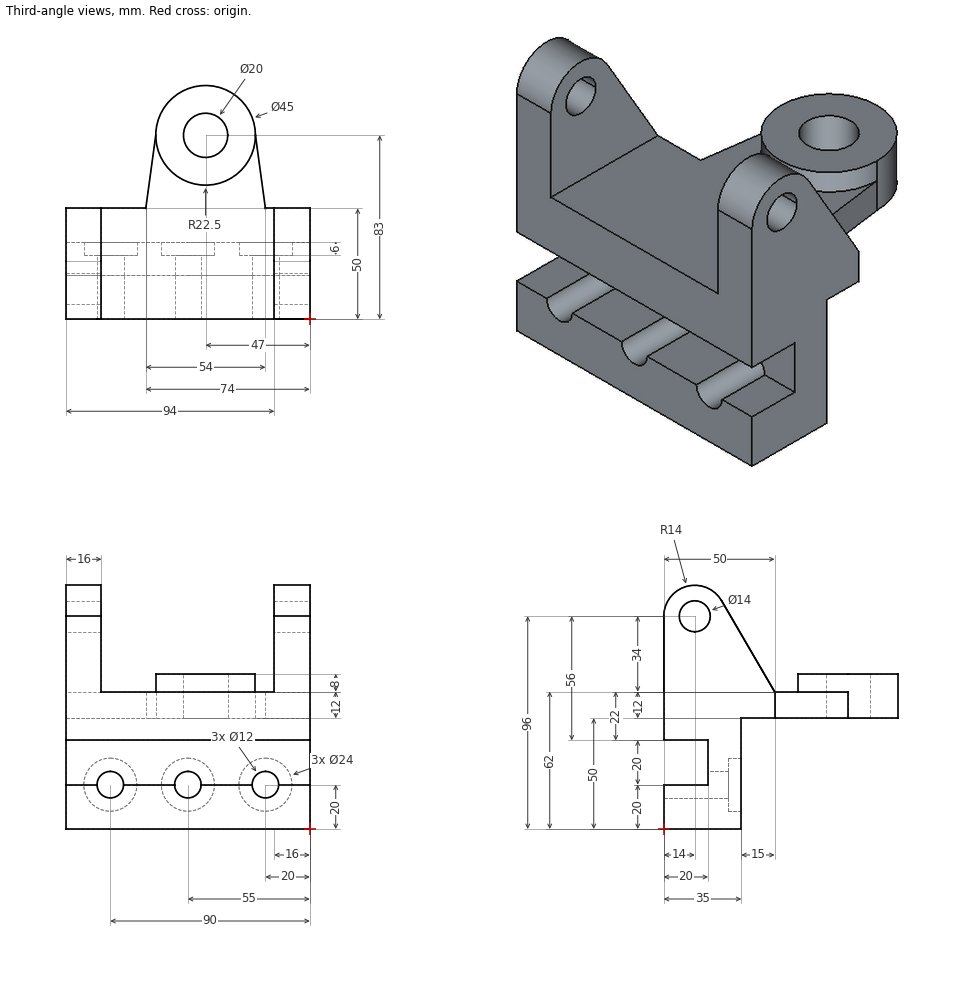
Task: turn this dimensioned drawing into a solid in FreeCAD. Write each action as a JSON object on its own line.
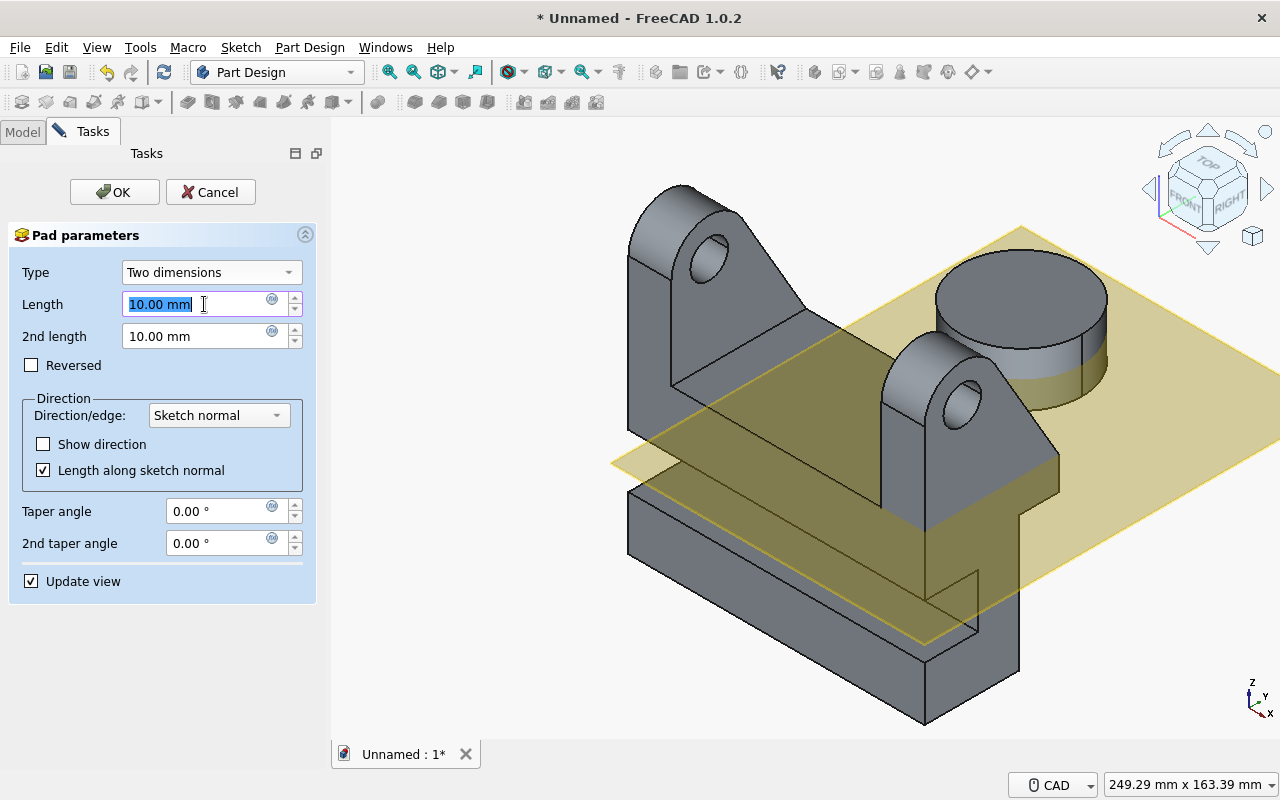
{"action": "type", "text": "8"}
{"action": "key", "text": "Tab"}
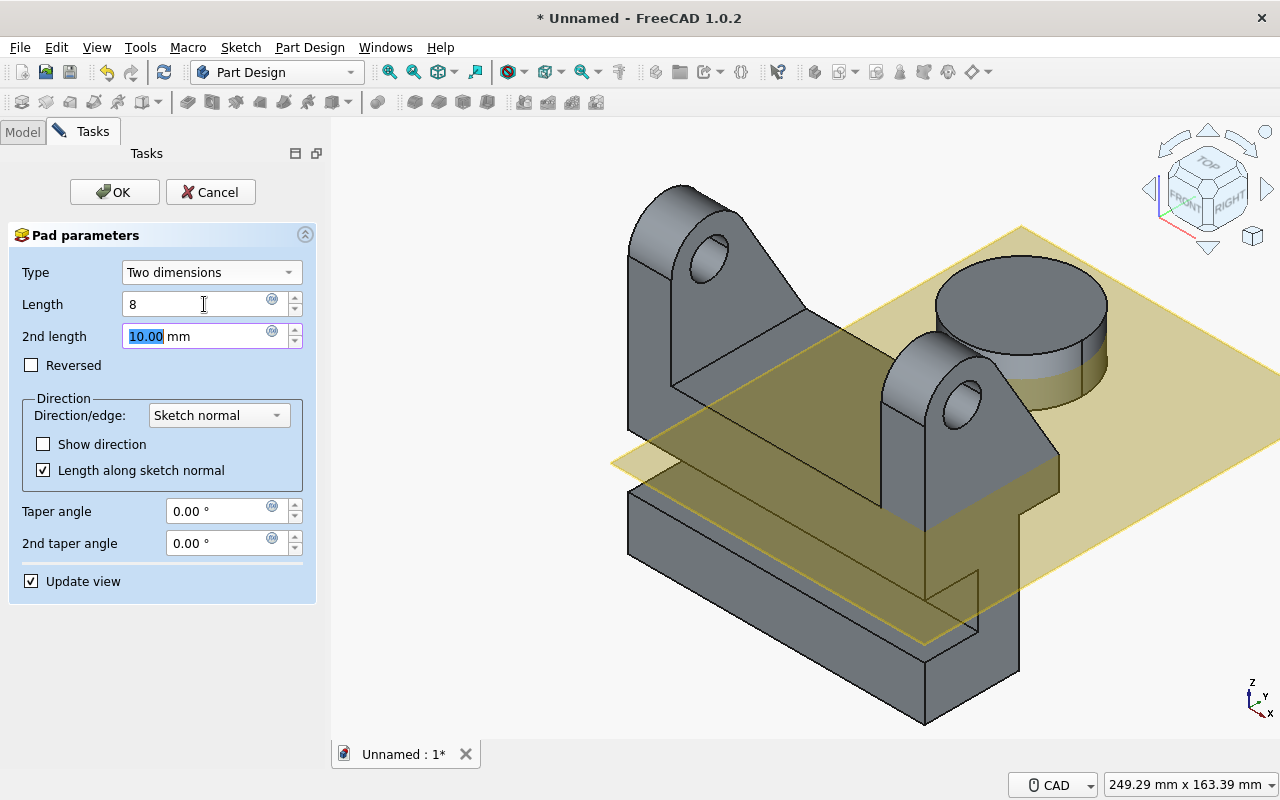
{"action": "type", "text": "12"}
{"action": "key", "text": "Tab"}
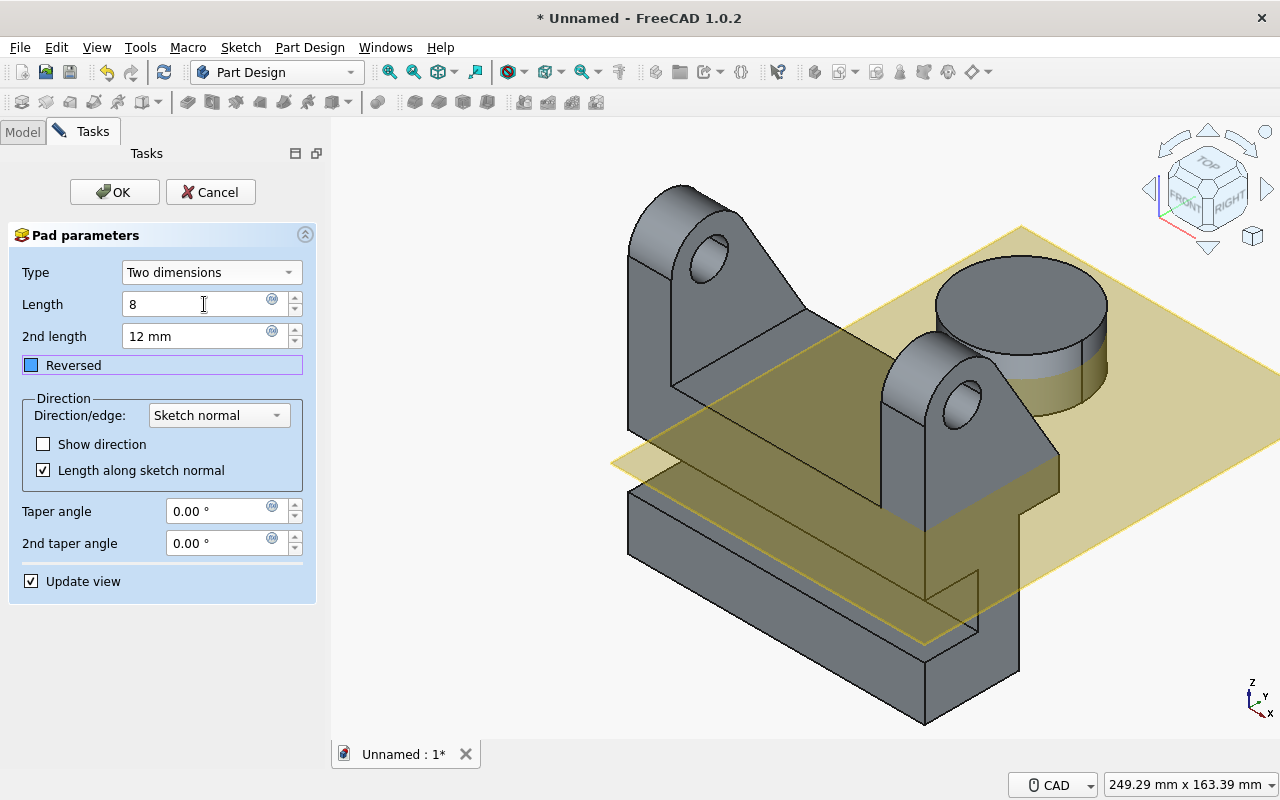
{"action": "left_click", "coordinate": [115, 192]}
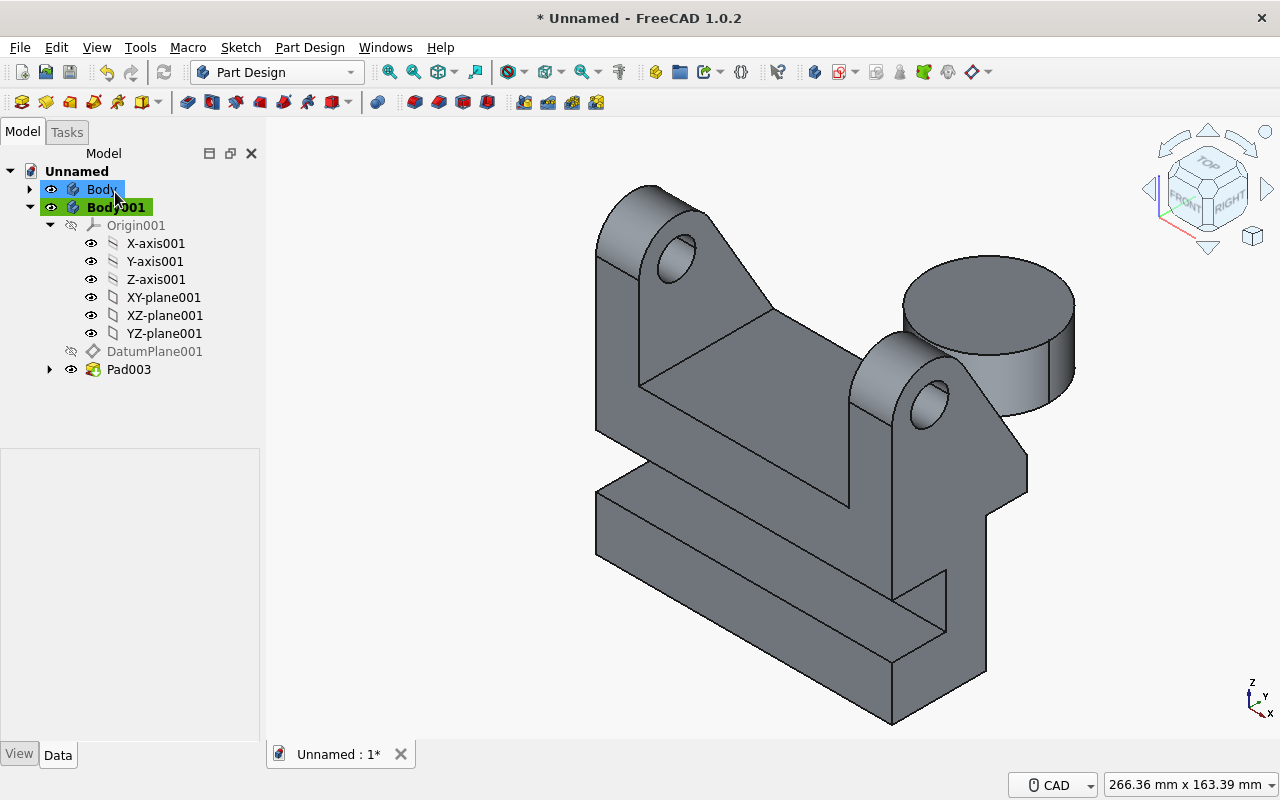
{"action": "left_click", "coordinate": [390, 72]}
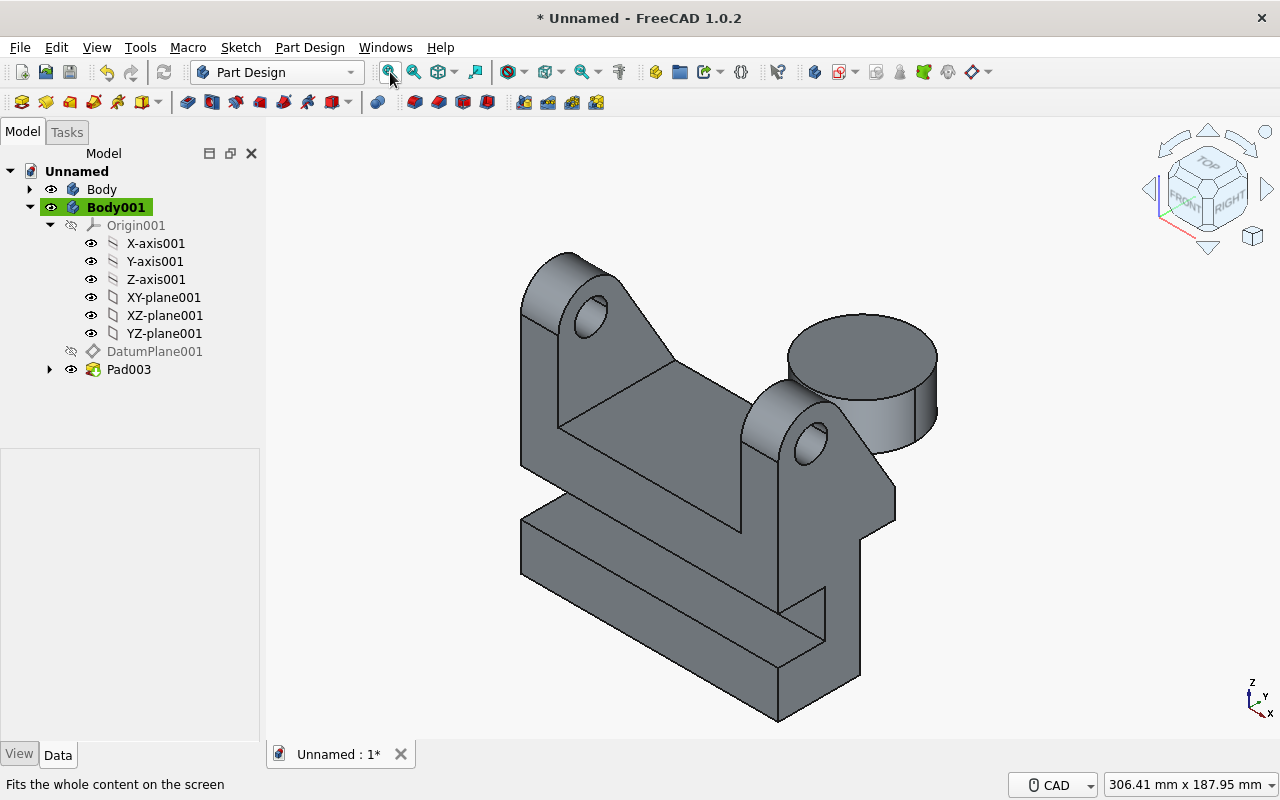
{"action": "double_click", "coordinate": [96, 189]}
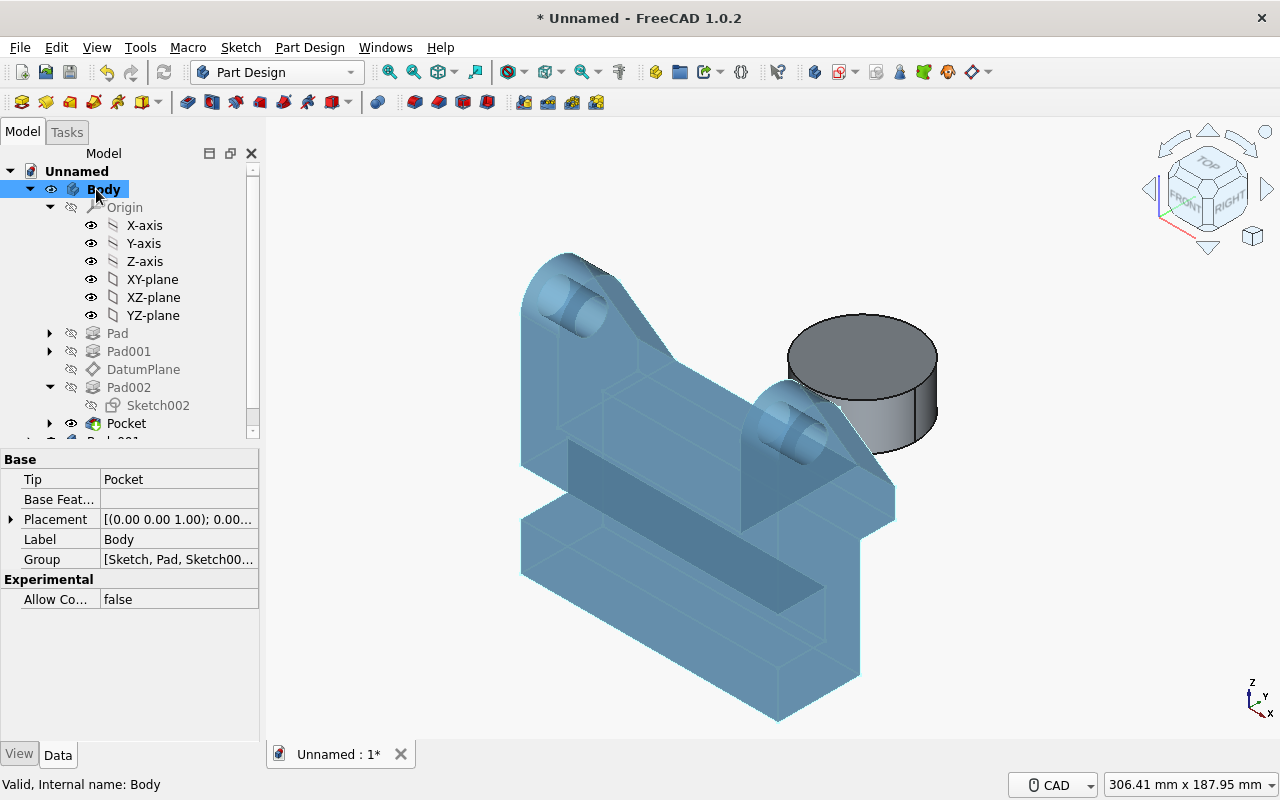
{"action": "left_click", "coordinate": [96, 189]}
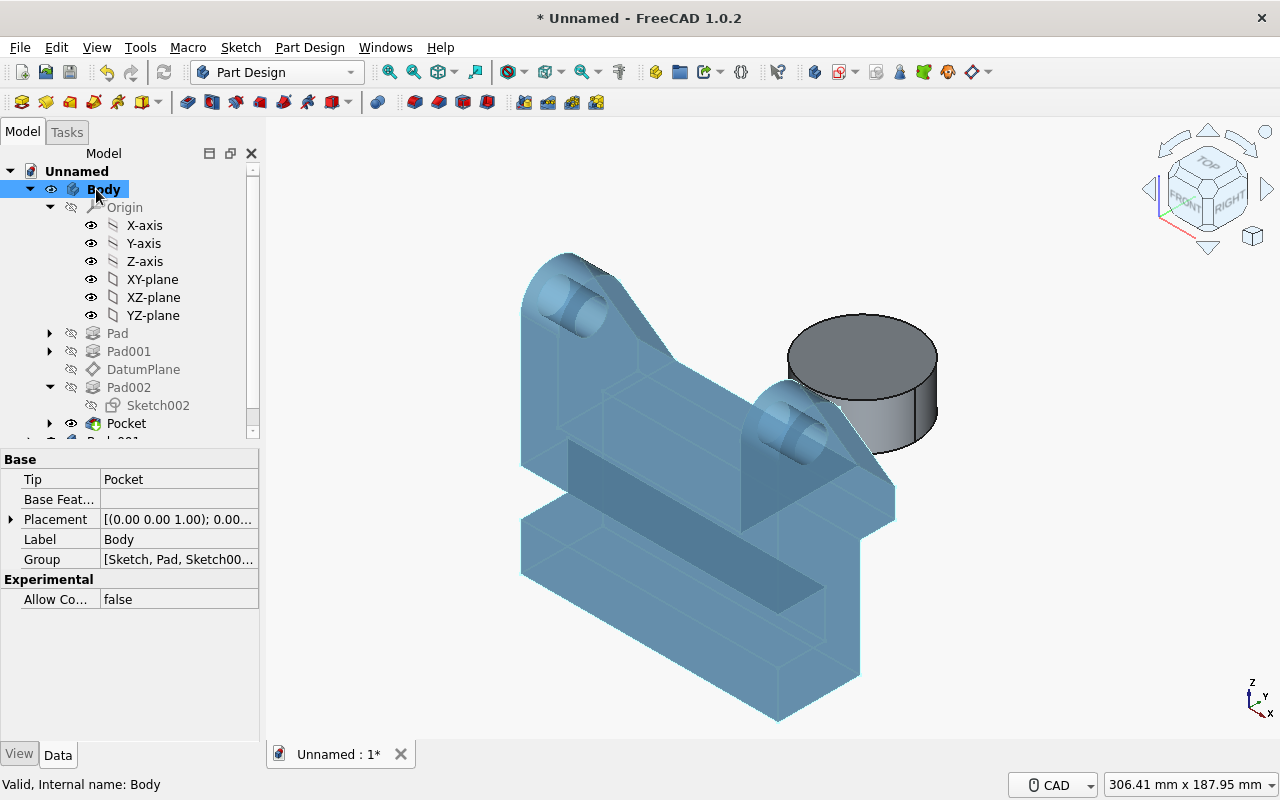
{"action": "left_click", "coordinate": [146, 599]}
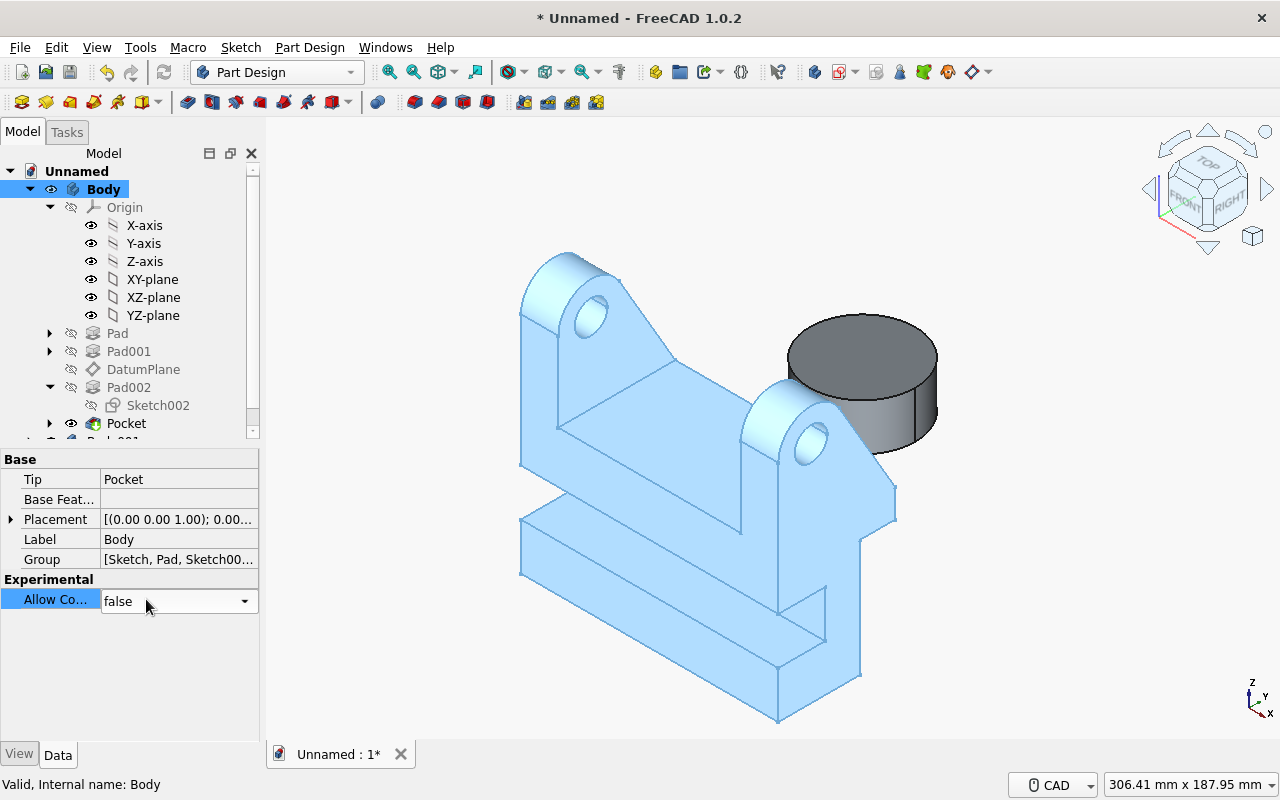
{"action": "left_click", "coordinate": [146, 599]}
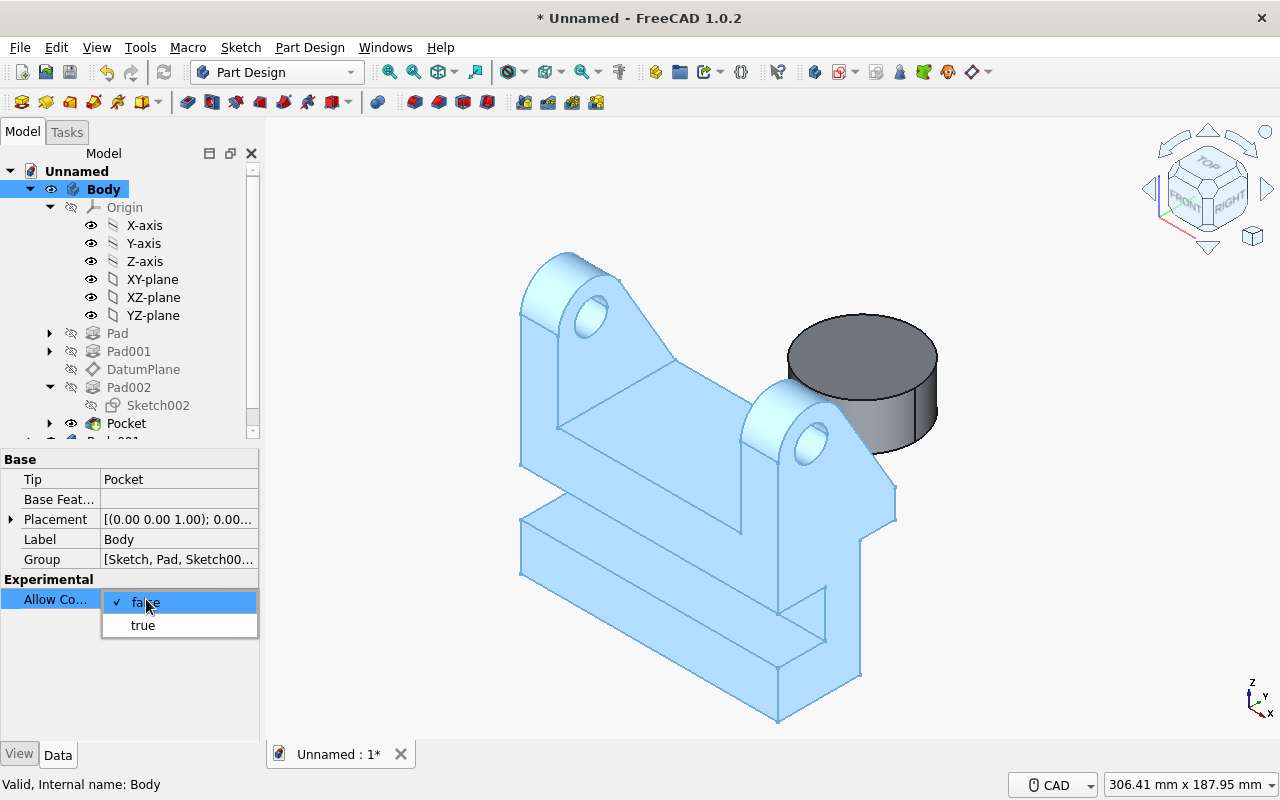
{"action": "left_click", "coordinate": [179, 626]}
{"action": "key", "text": "Return"}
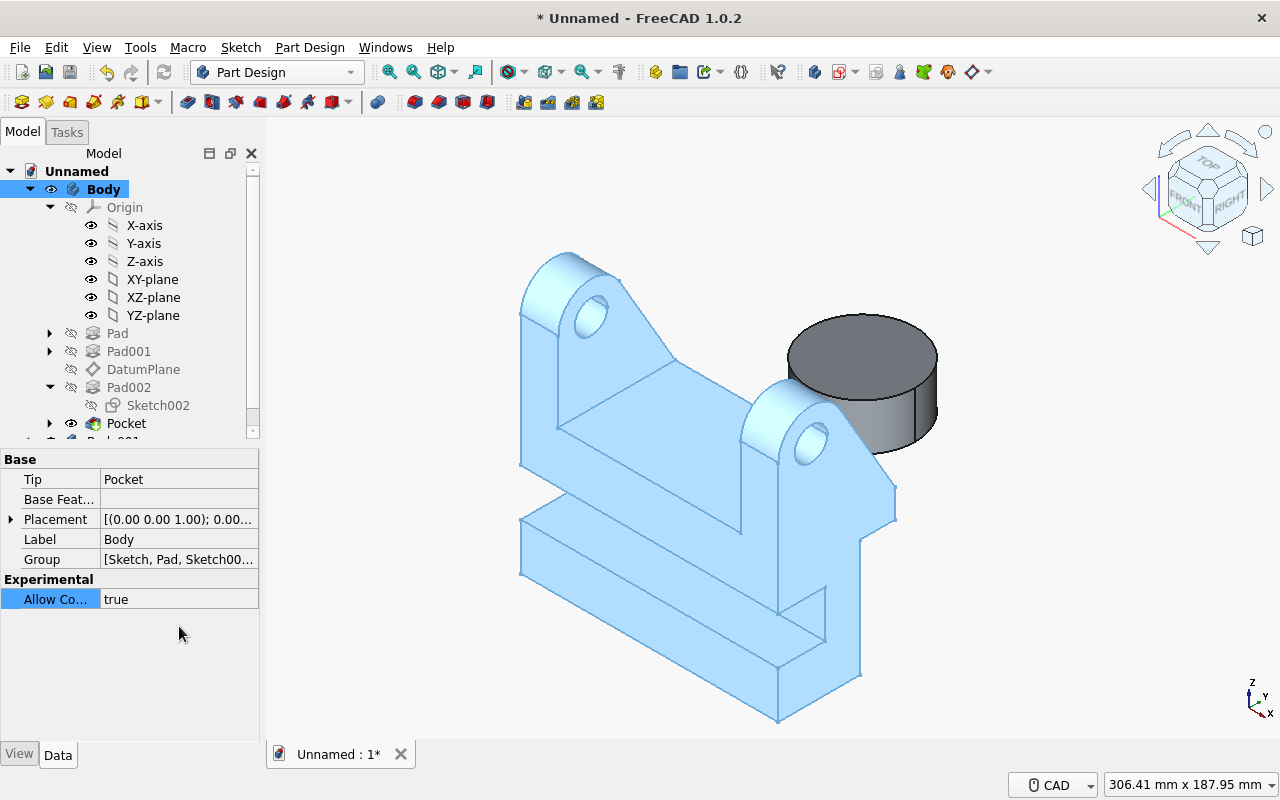
{"action": "scroll", "coordinate": [100, 293], "scroll_direction": "down", "scroll_amount": 3}